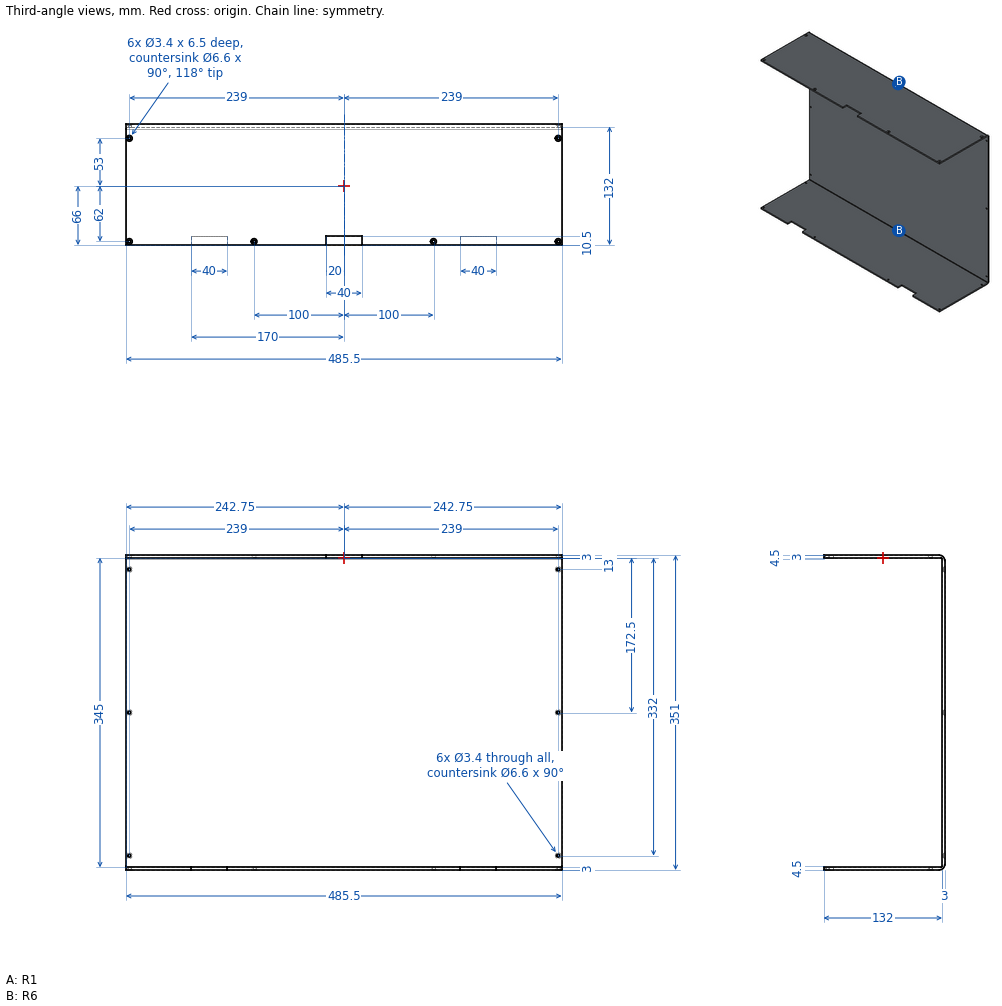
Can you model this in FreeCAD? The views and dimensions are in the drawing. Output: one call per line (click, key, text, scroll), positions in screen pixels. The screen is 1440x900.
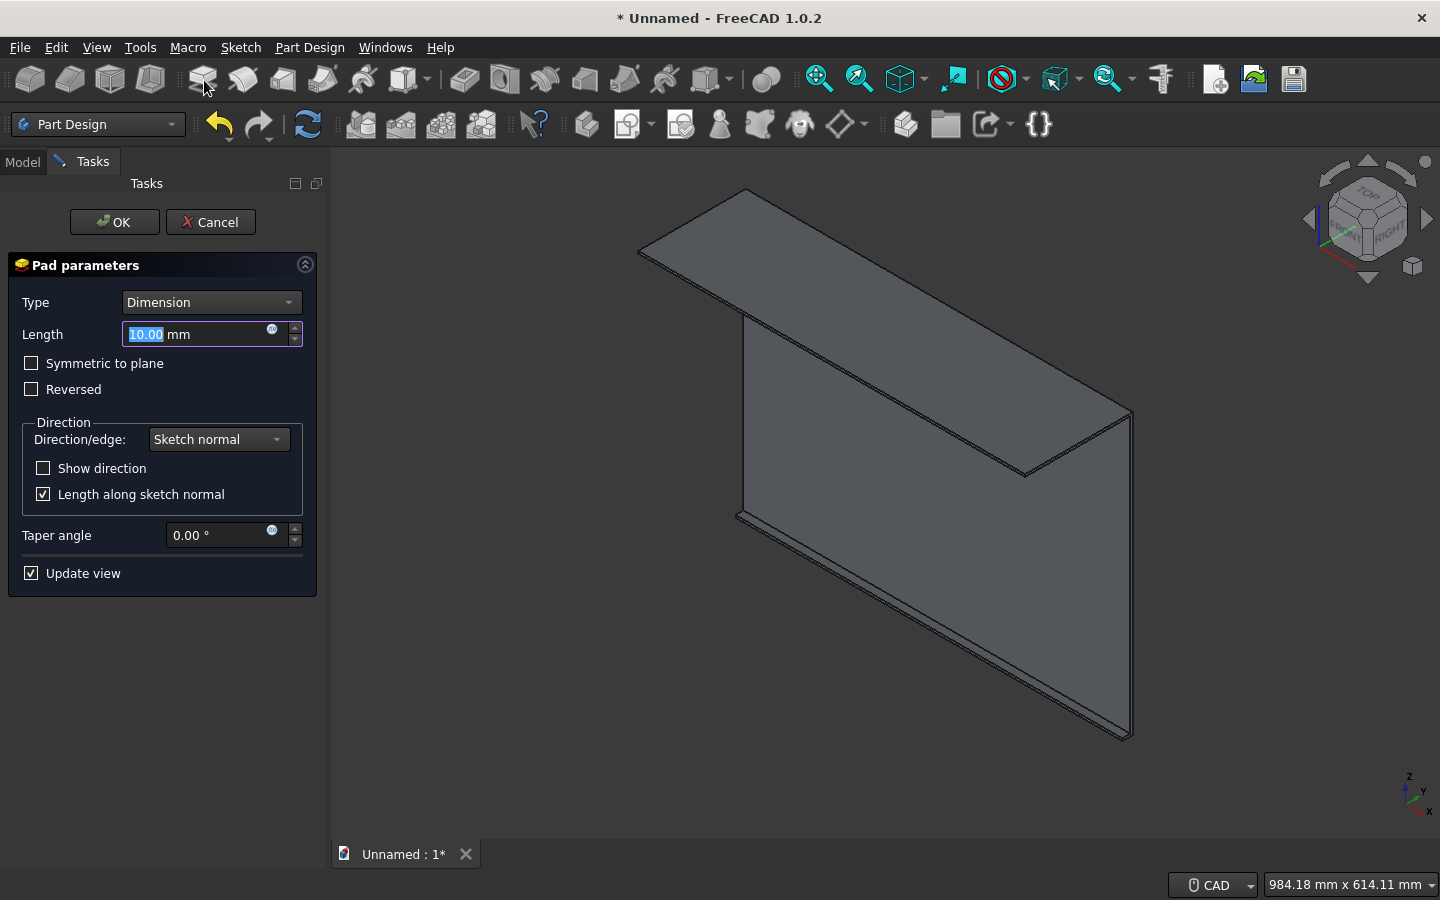
text(132)
key(Tab)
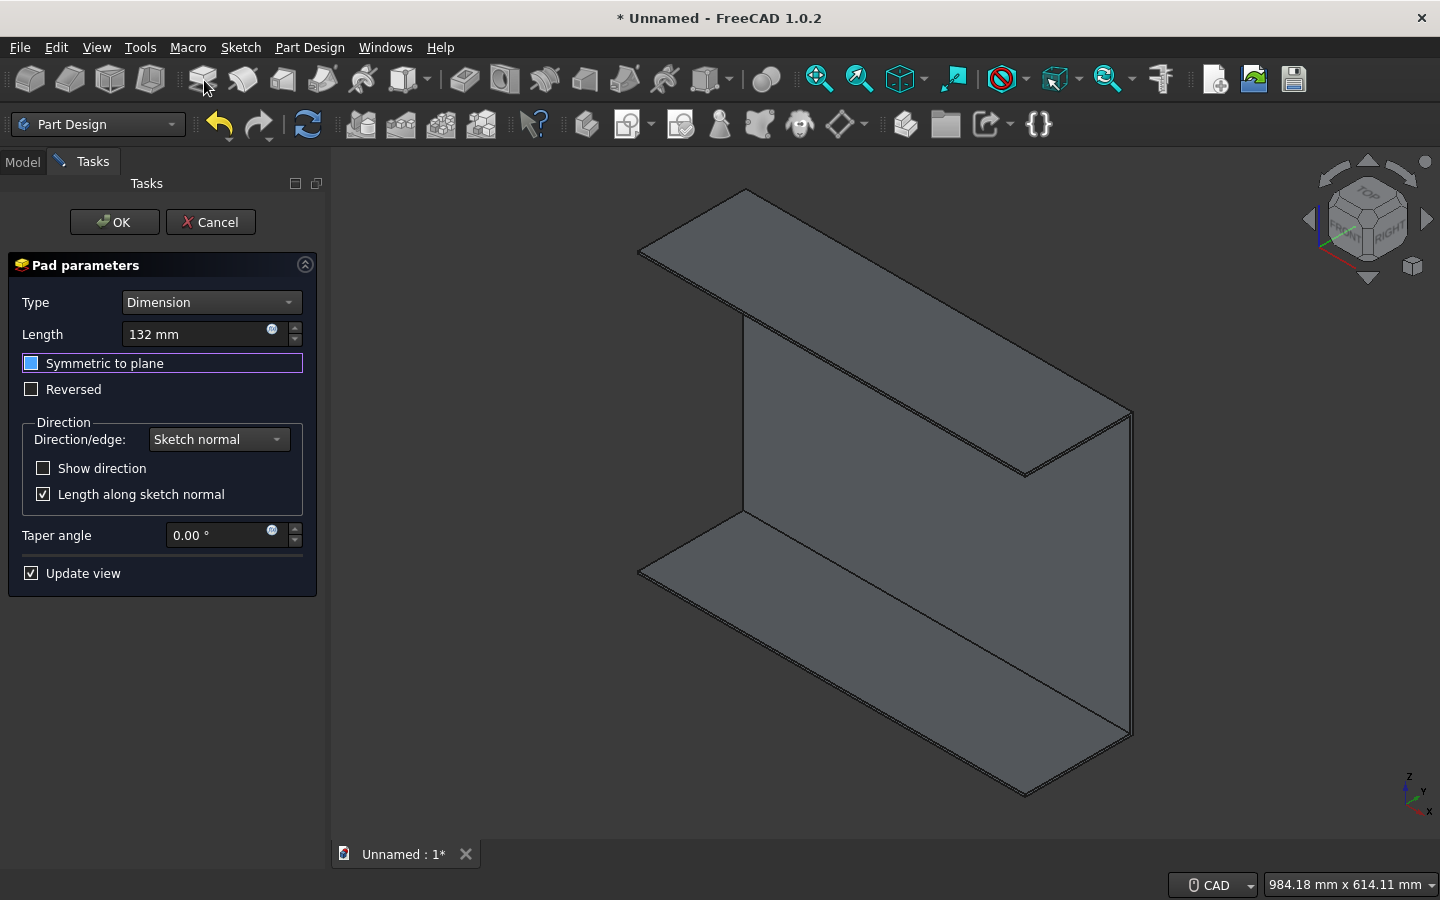
click(115, 222)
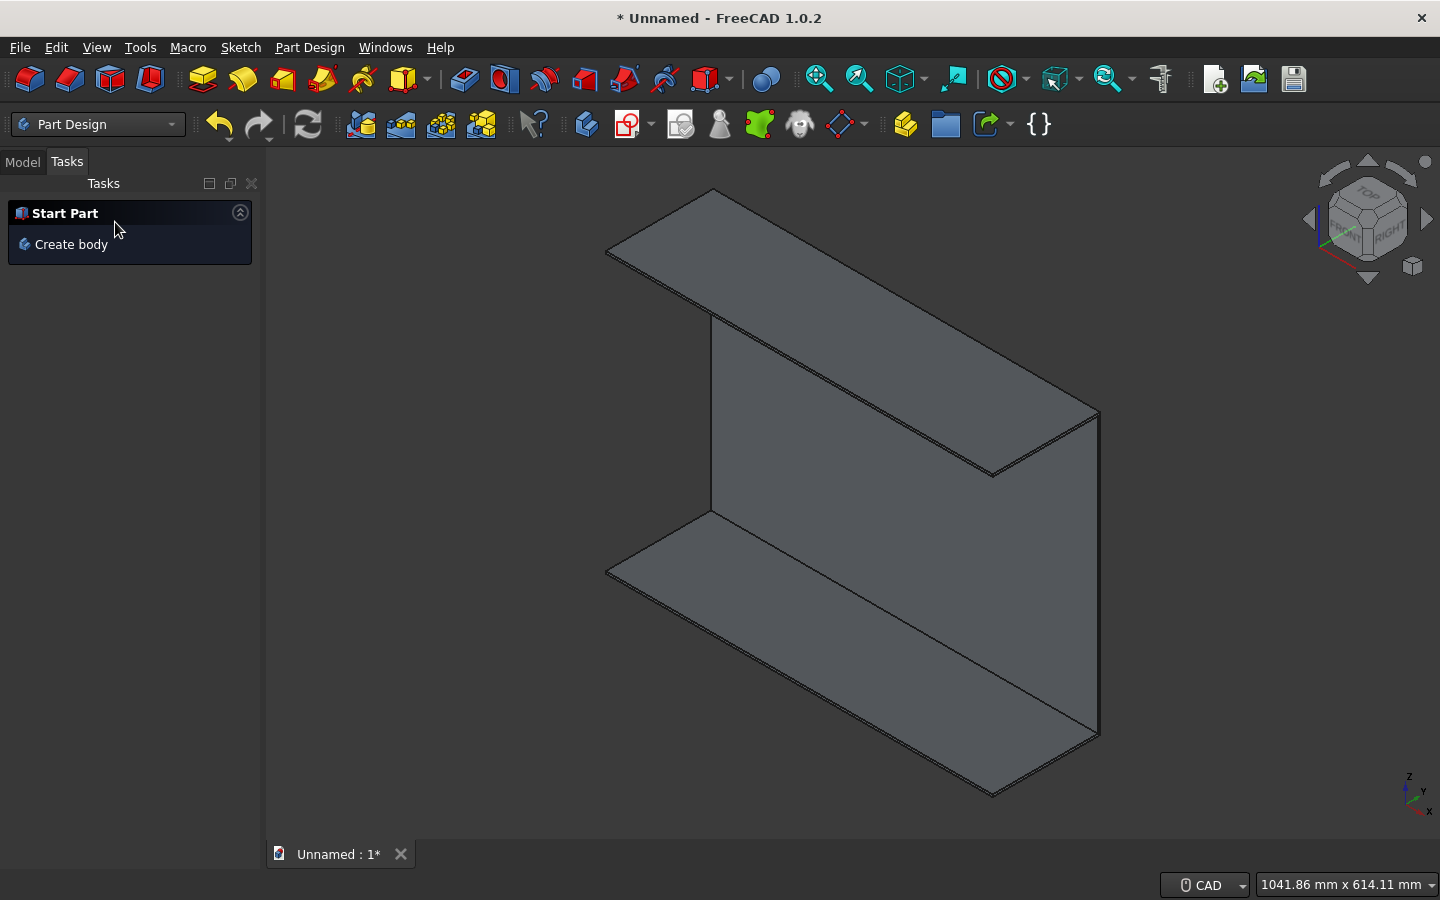
key(2)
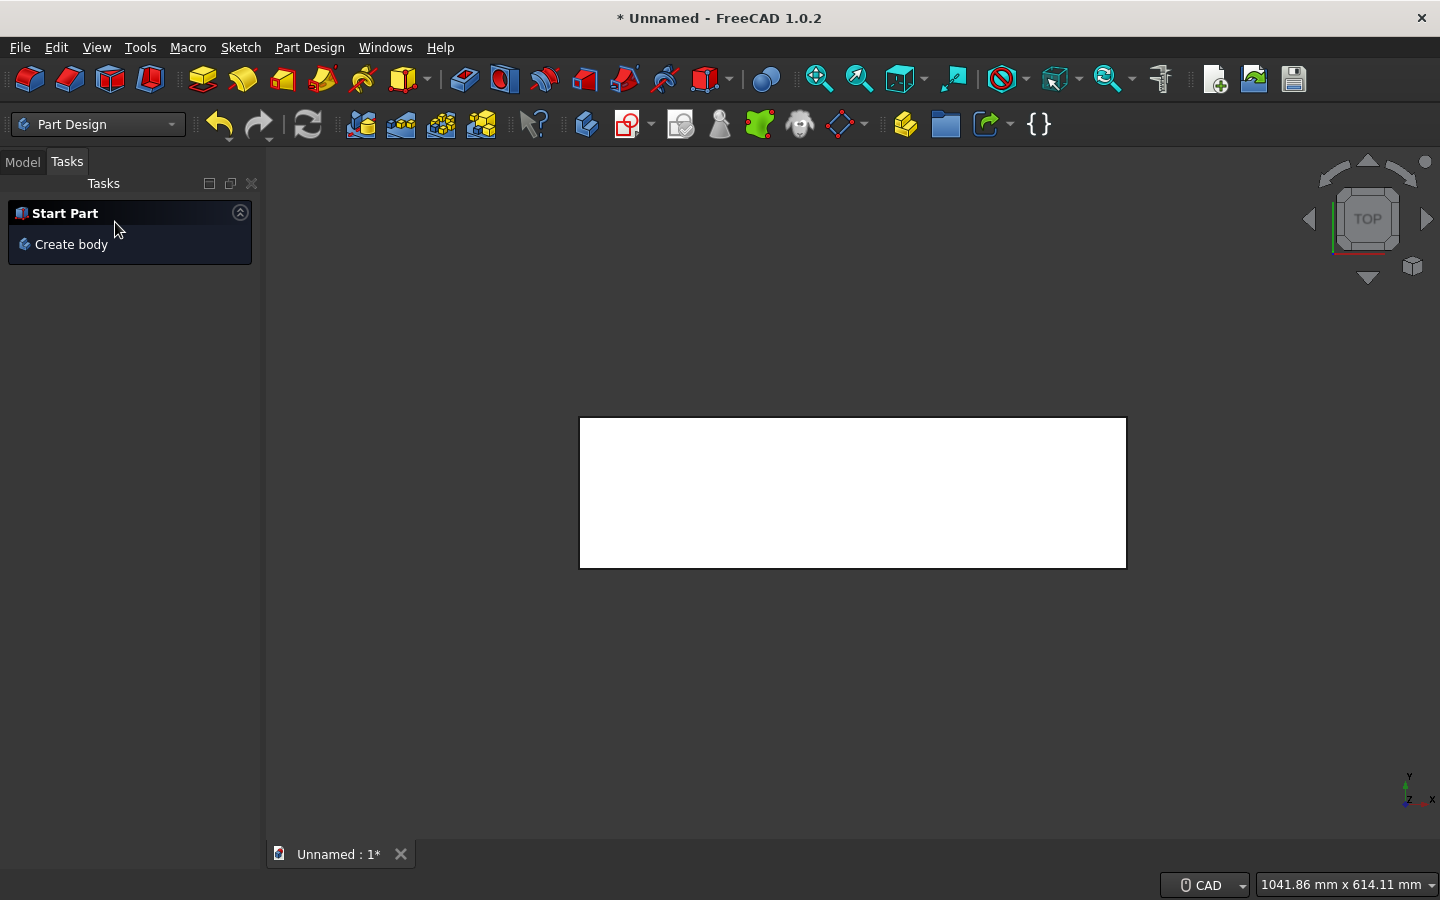
key(0)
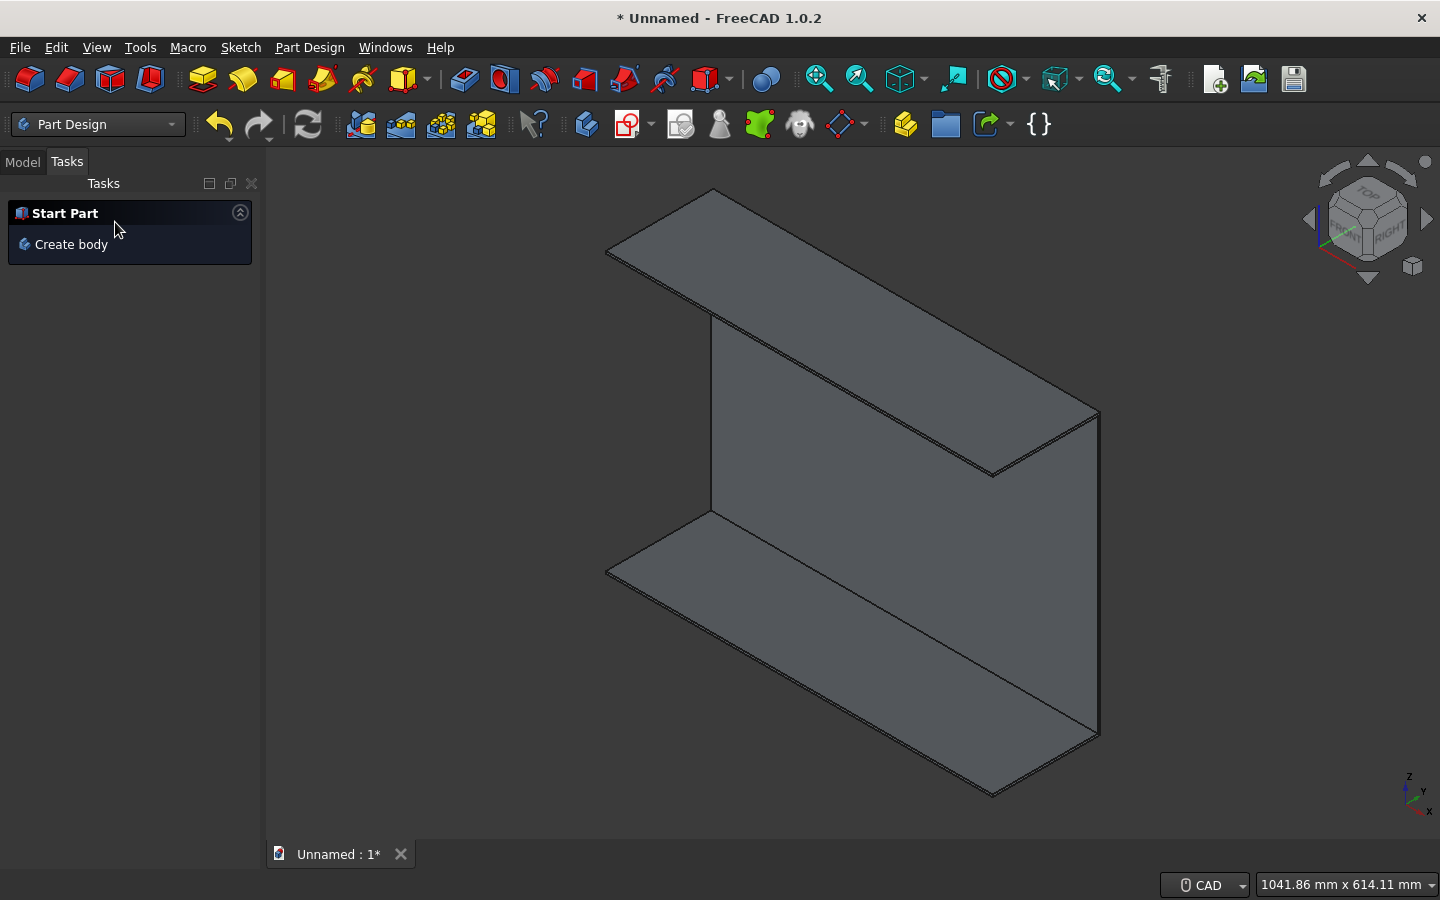
key(1)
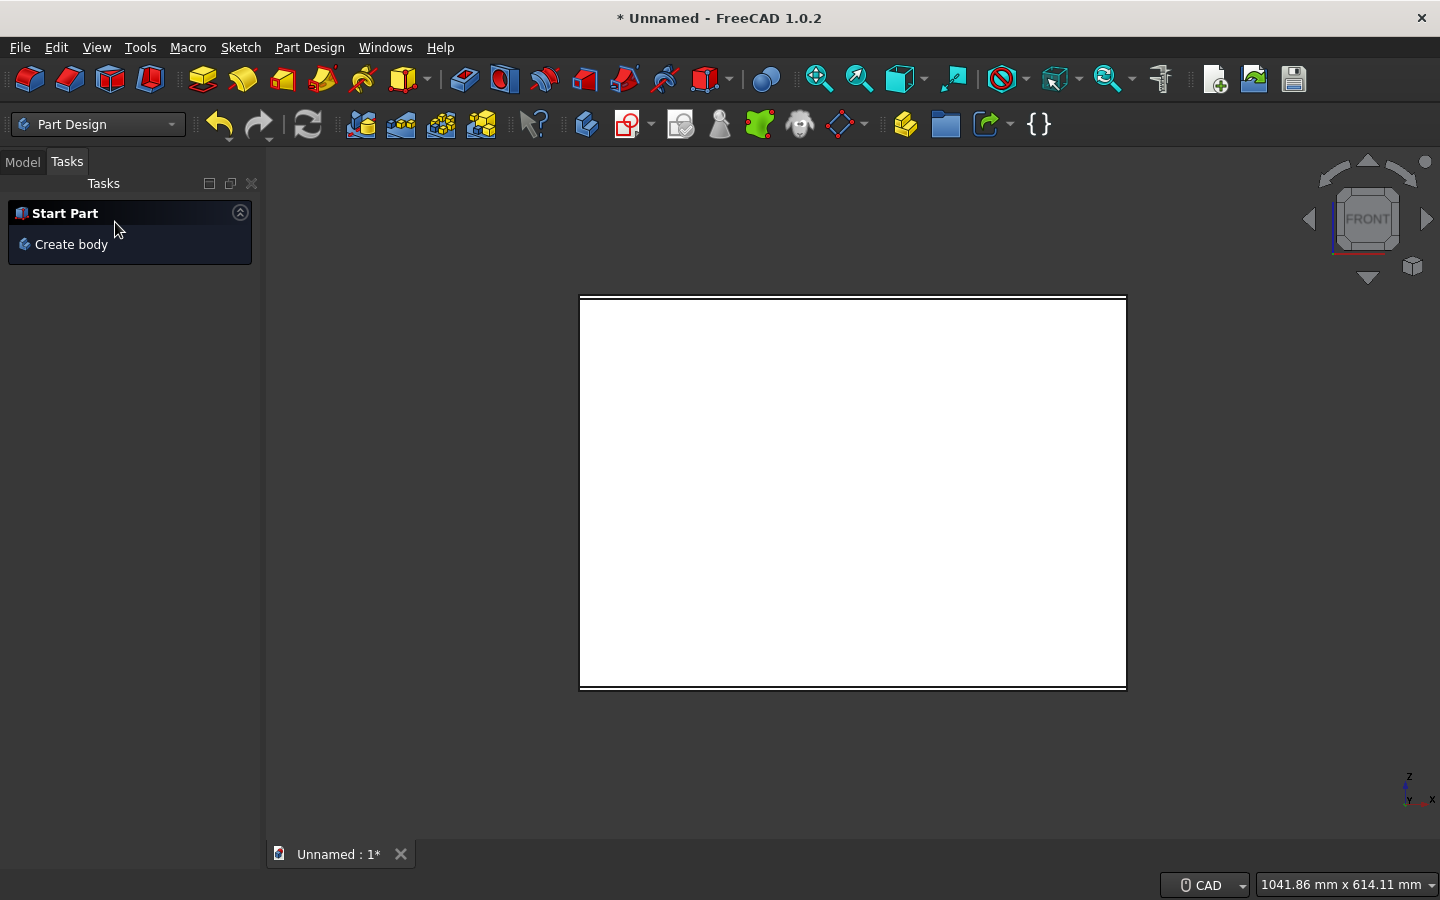
key(3)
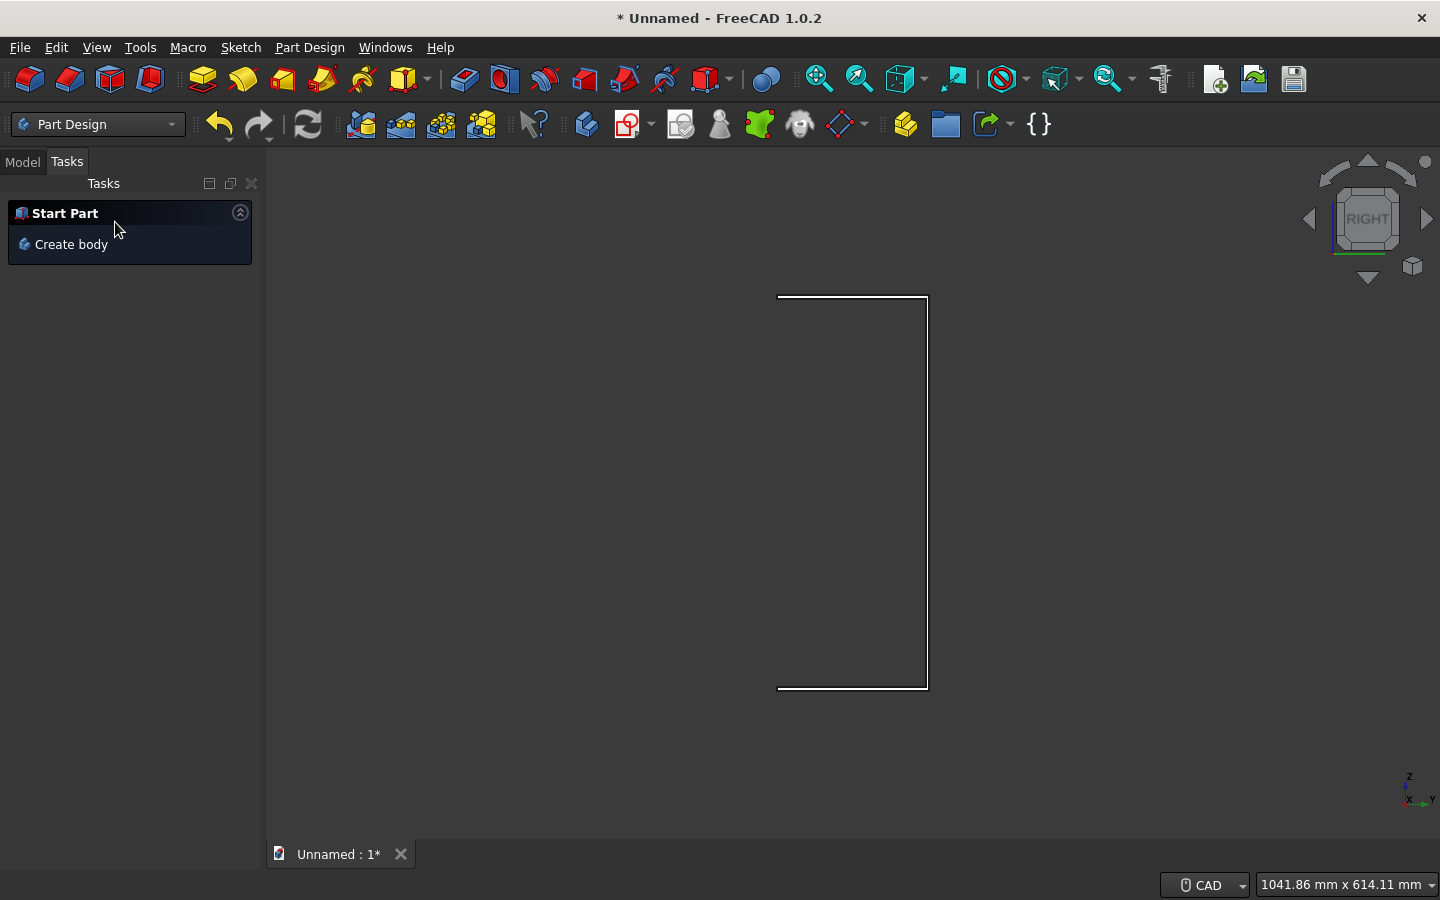
key(5)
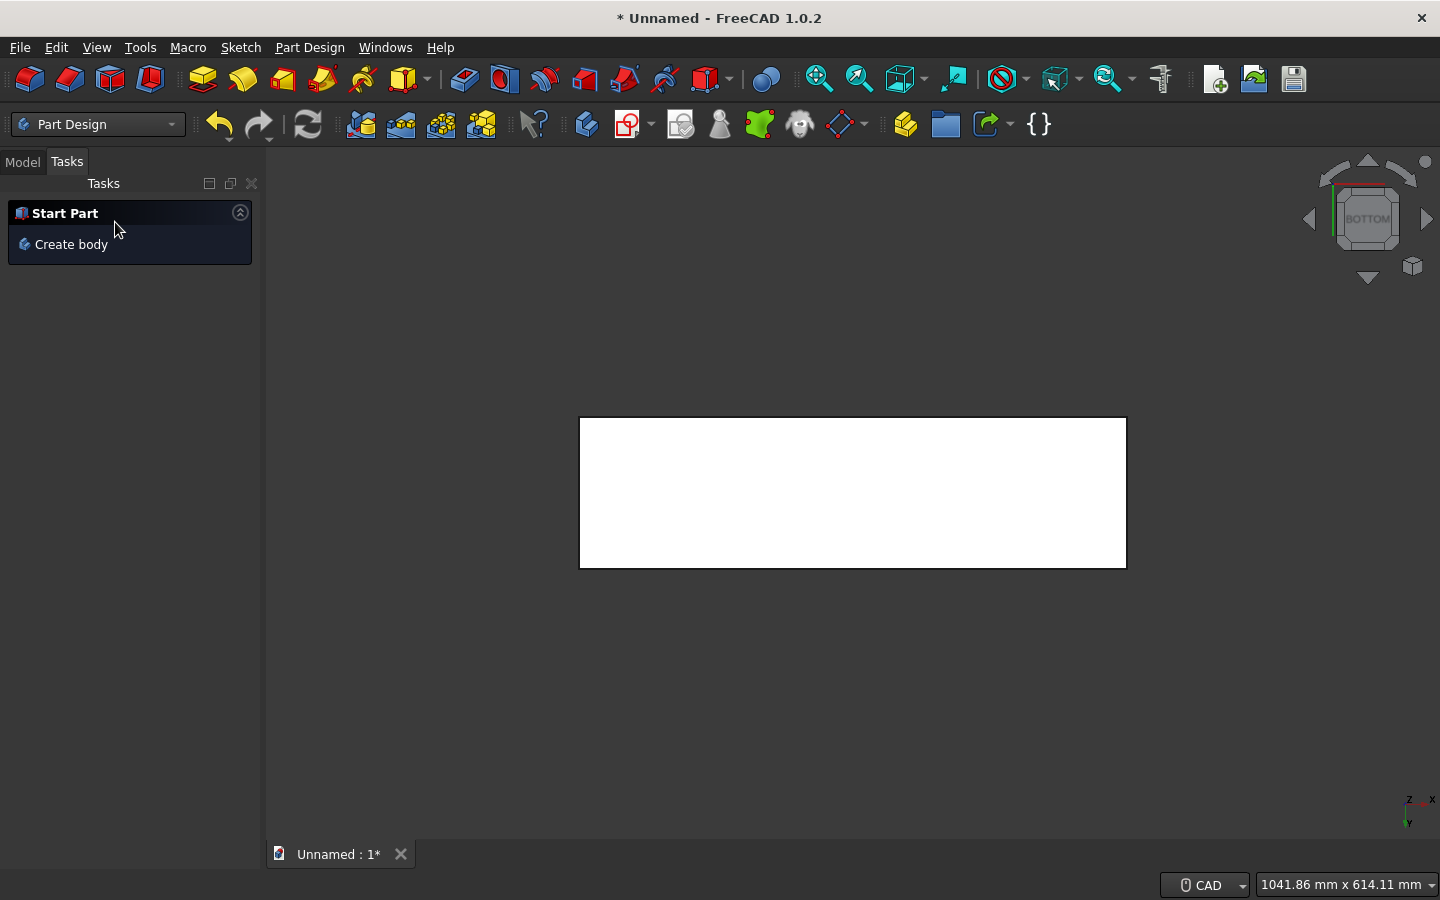
key(4)